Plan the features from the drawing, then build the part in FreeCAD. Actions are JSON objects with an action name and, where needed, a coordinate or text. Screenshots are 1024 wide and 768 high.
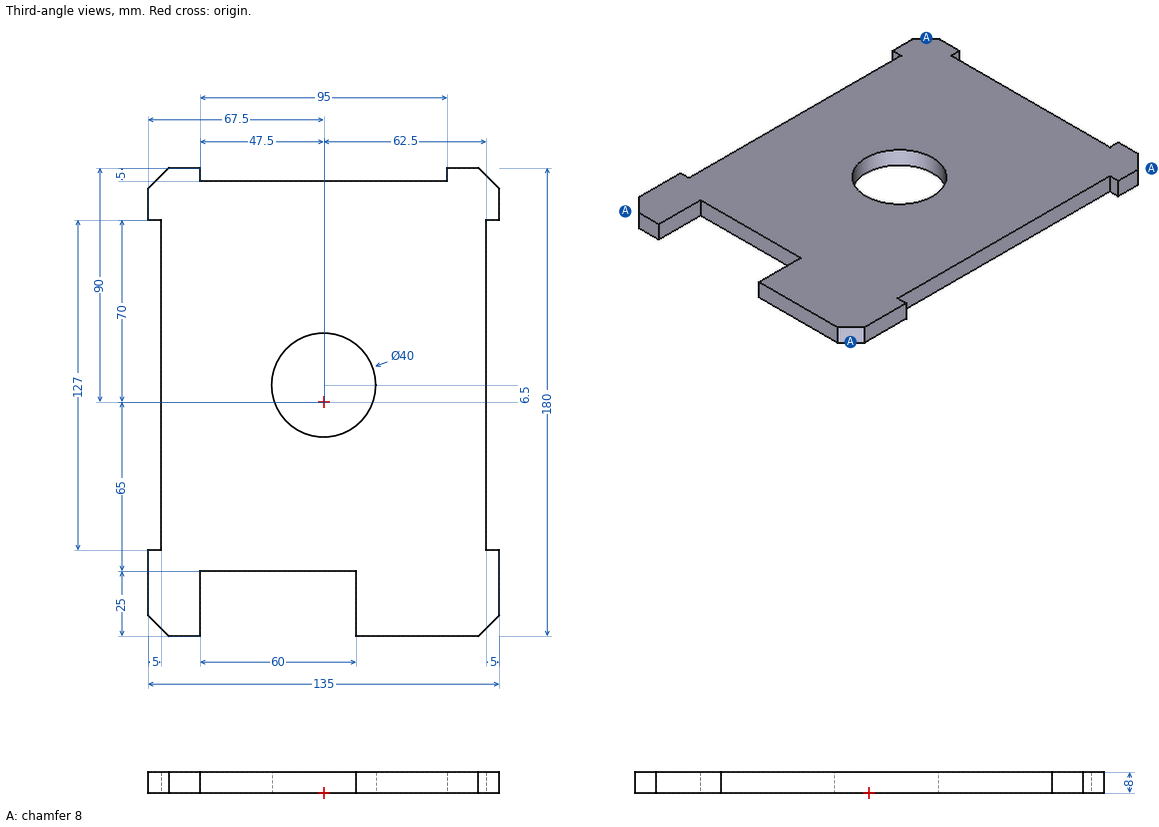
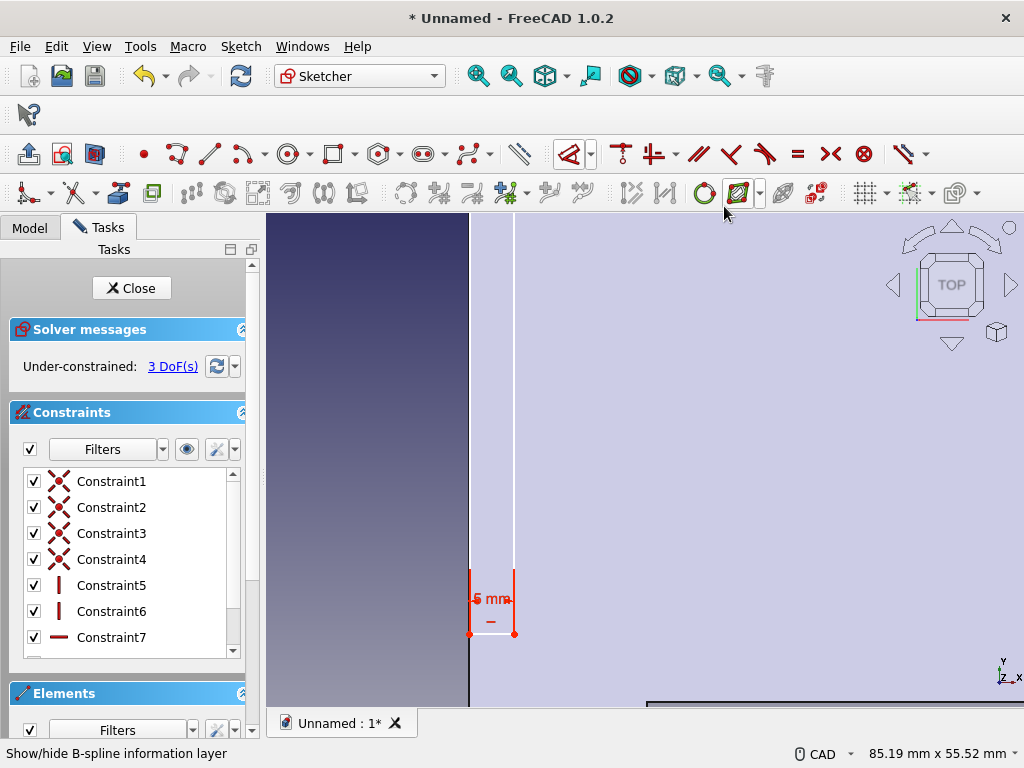
{"action": "scroll", "coordinate": [493, 630], "scroll_direction": "down", "scroll_amount": 6}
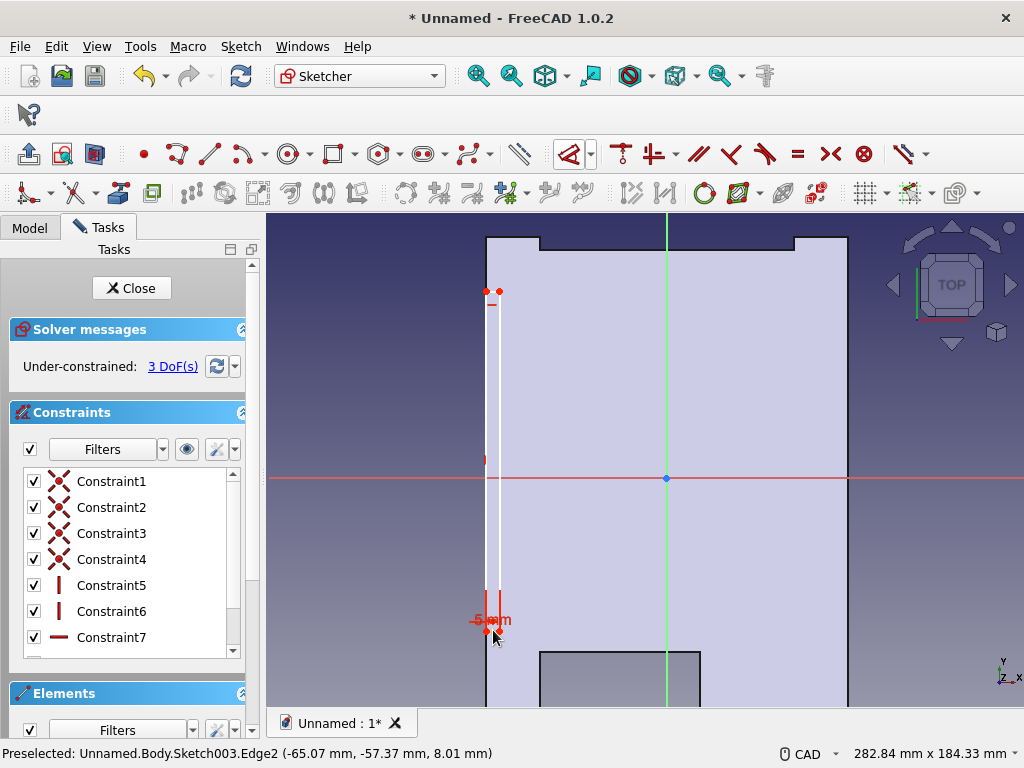
{"action": "left_click", "coordinate": [486, 530]}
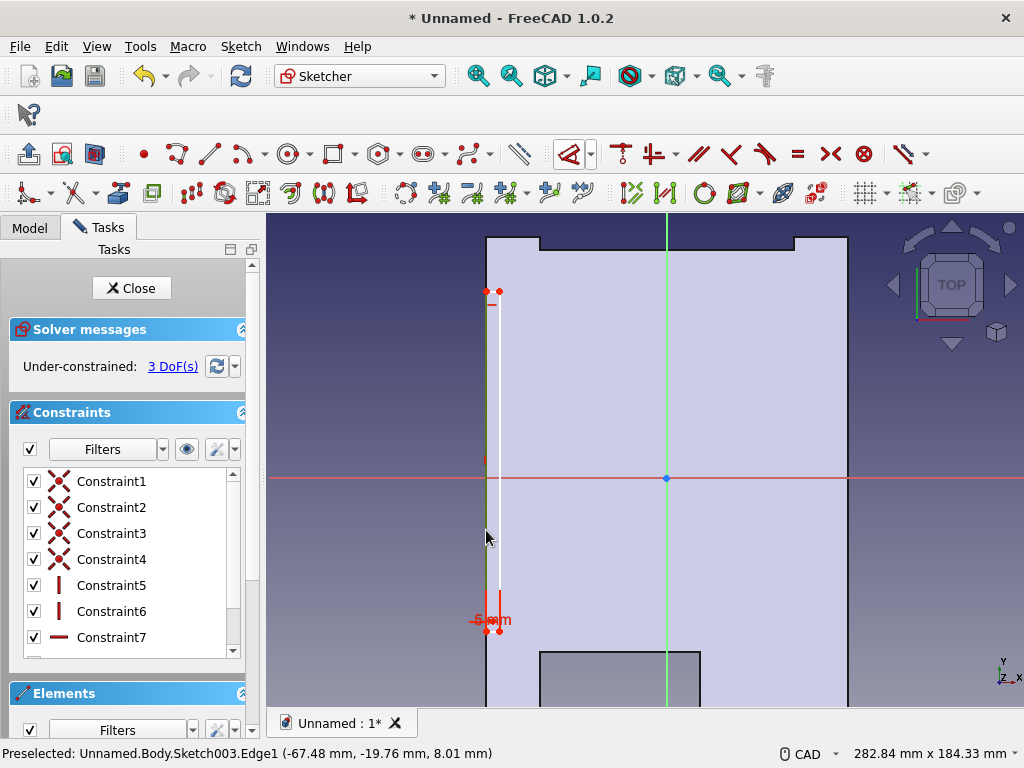
{"action": "key", "text": "i"}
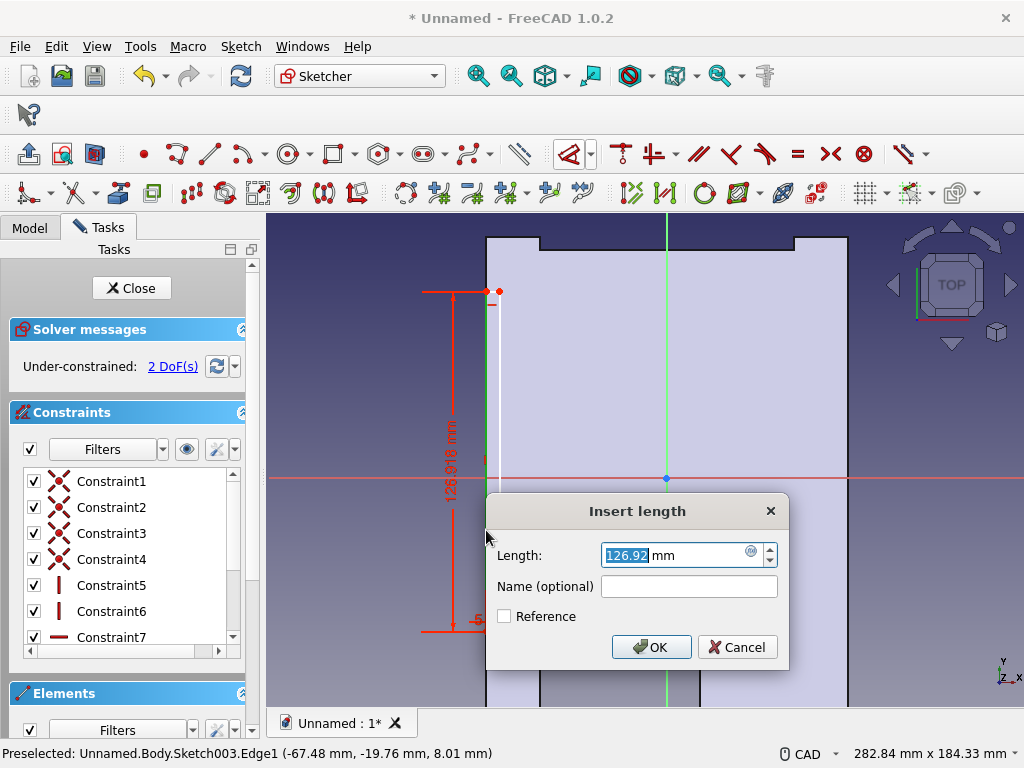
{"action": "type", "text": "127"}
{"action": "key", "text": "Return"}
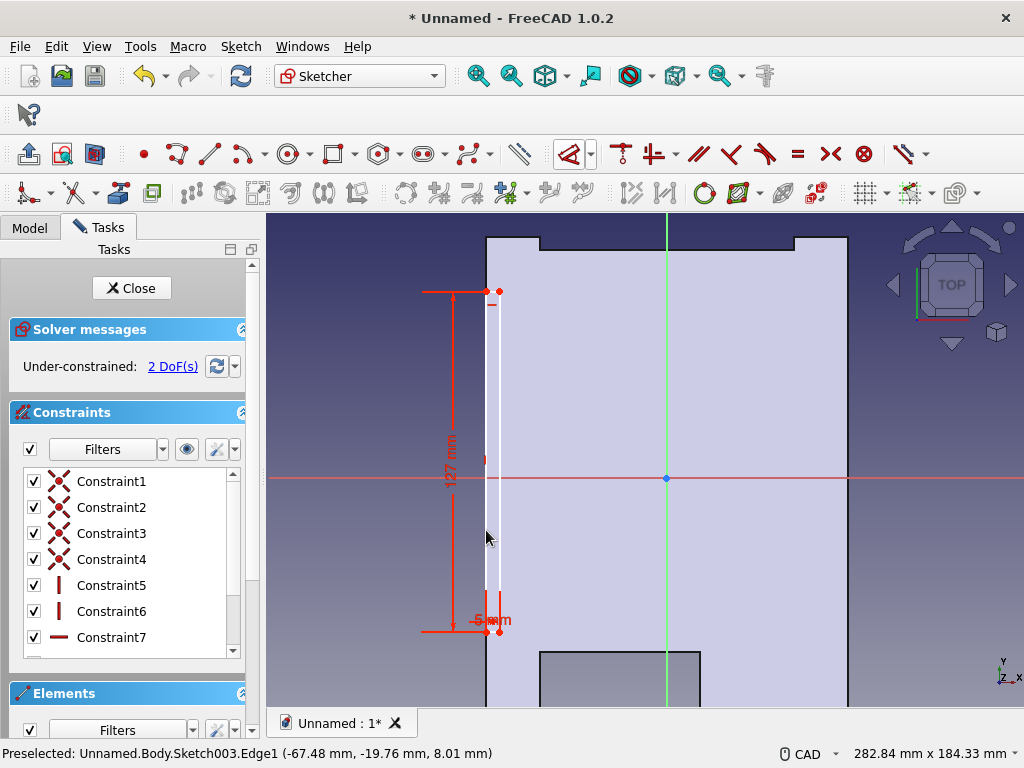
{"action": "left_click", "coordinate": [486, 292]}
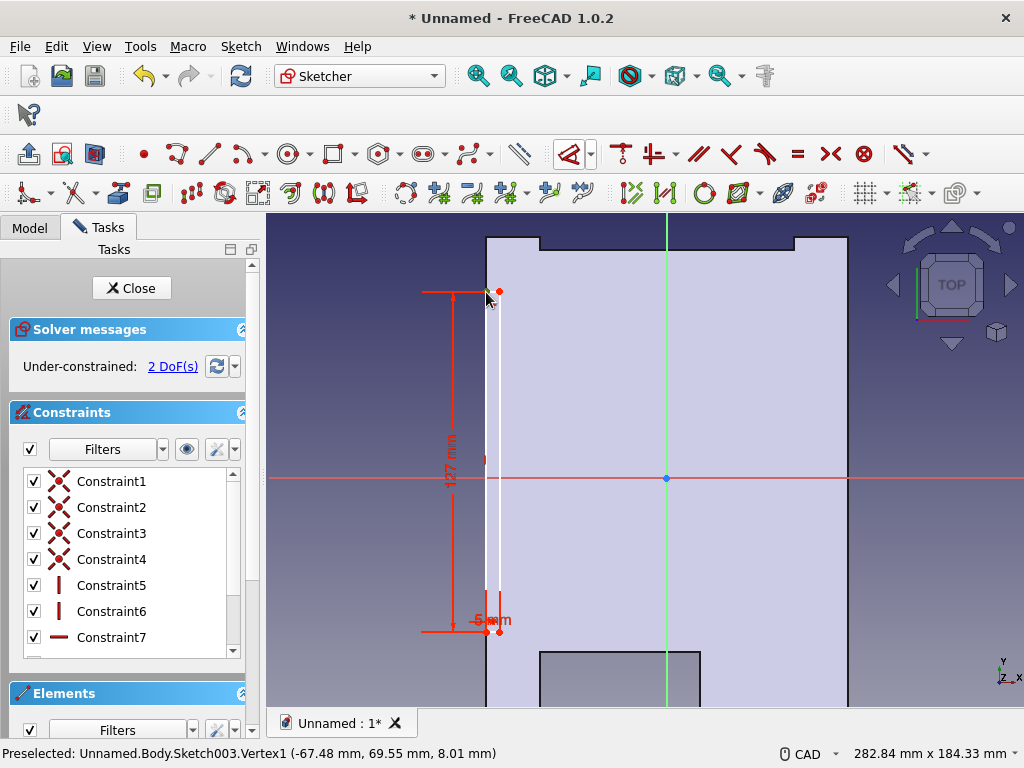
{"action": "left_click", "coordinate": [590, 154]}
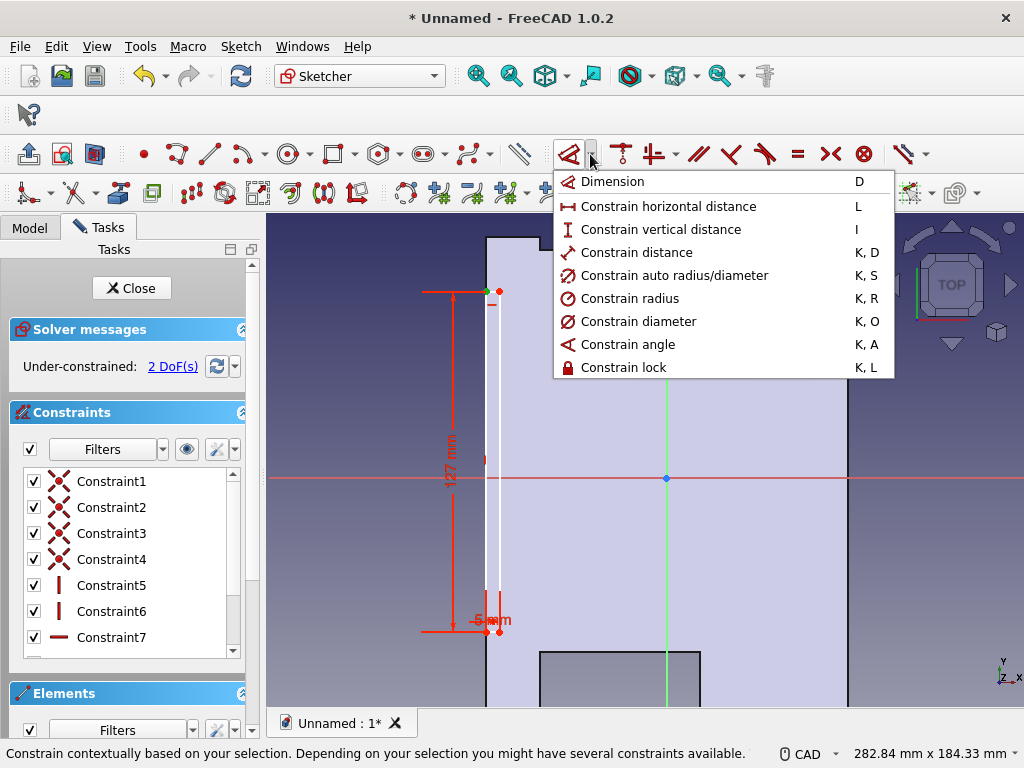
{"action": "left_click", "coordinate": [724, 230]}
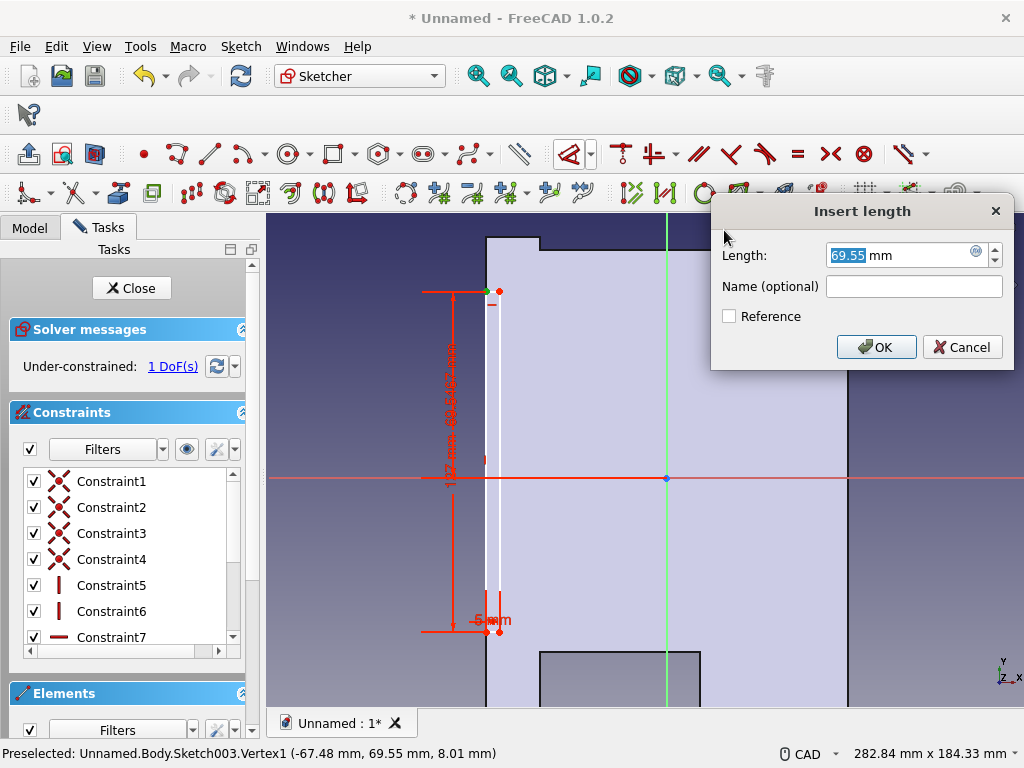
{"action": "type", "text": "70"}
{"action": "key", "text": "Return"}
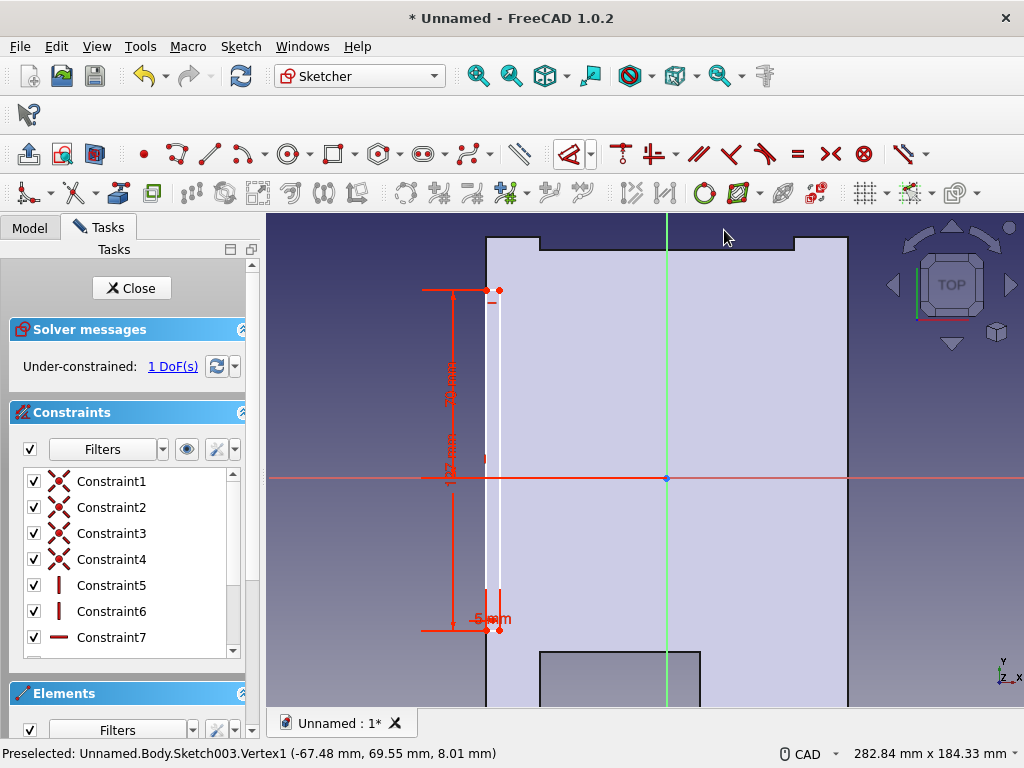
{"action": "left_click", "coordinate": [486, 290]}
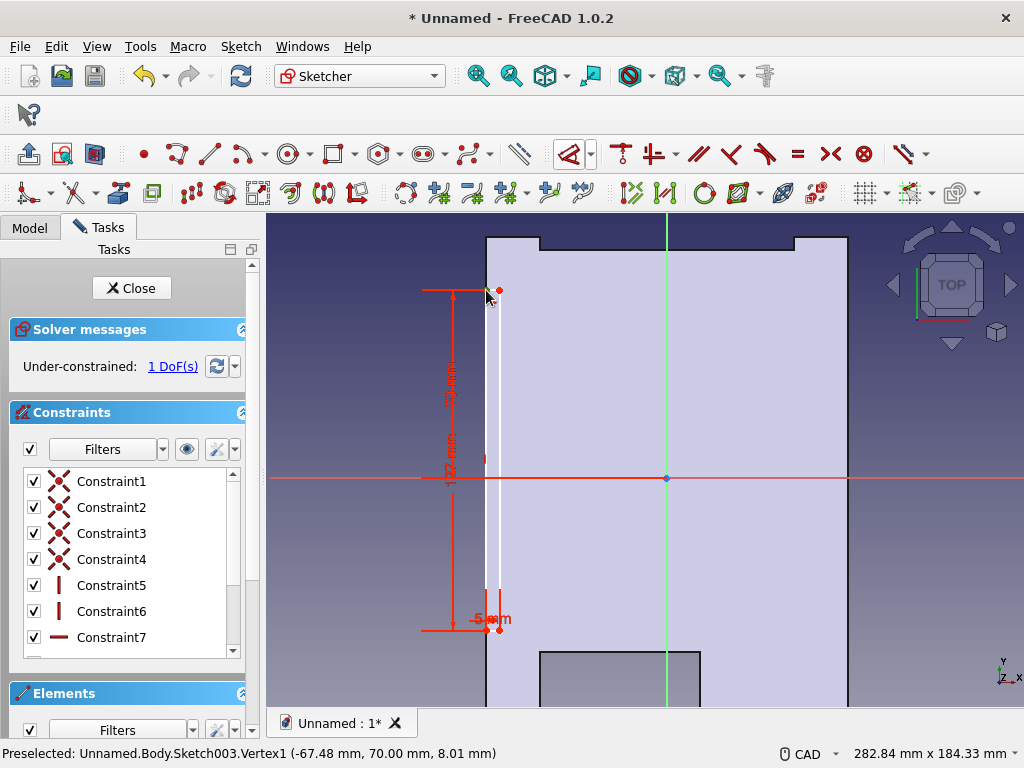
{"action": "key", "text": "l"}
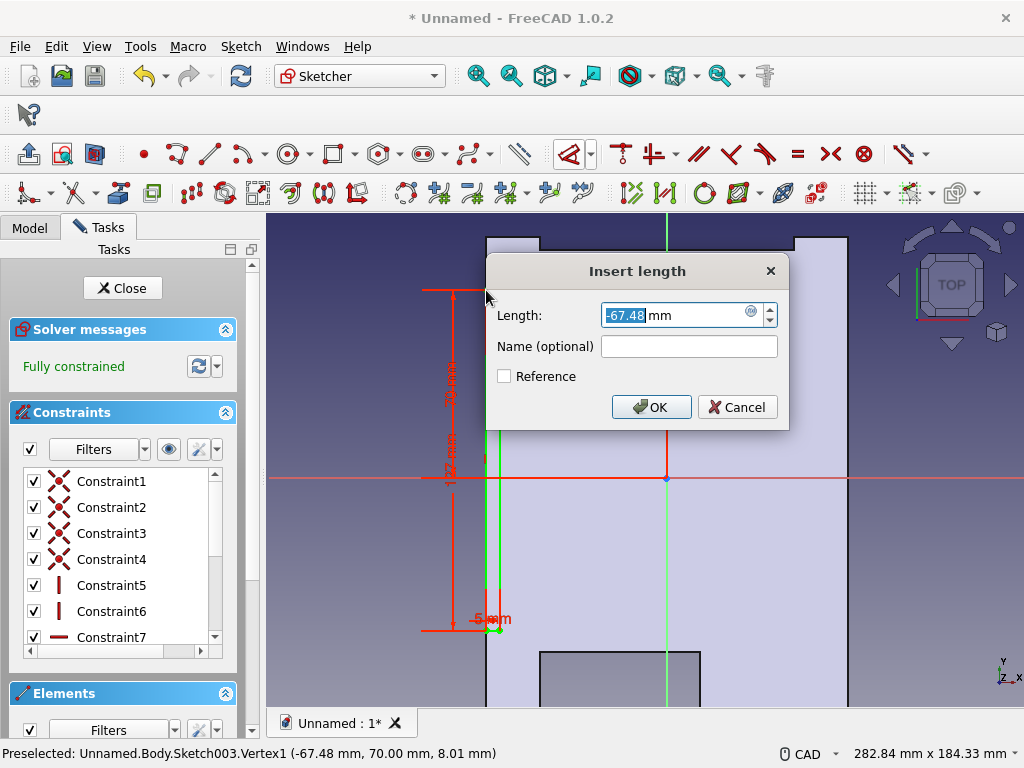
{"action": "type", "text": "-67.5"}
{"action": "key", "text": "Return"}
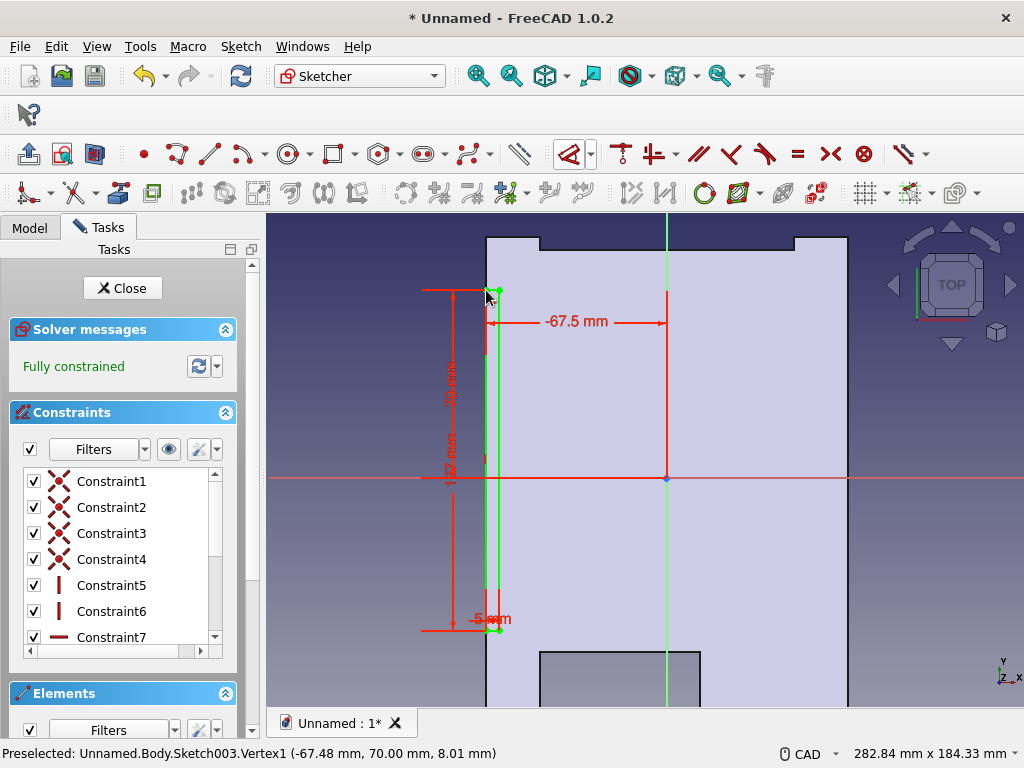
{"action": "left_click", "coordinate": [123, 288]}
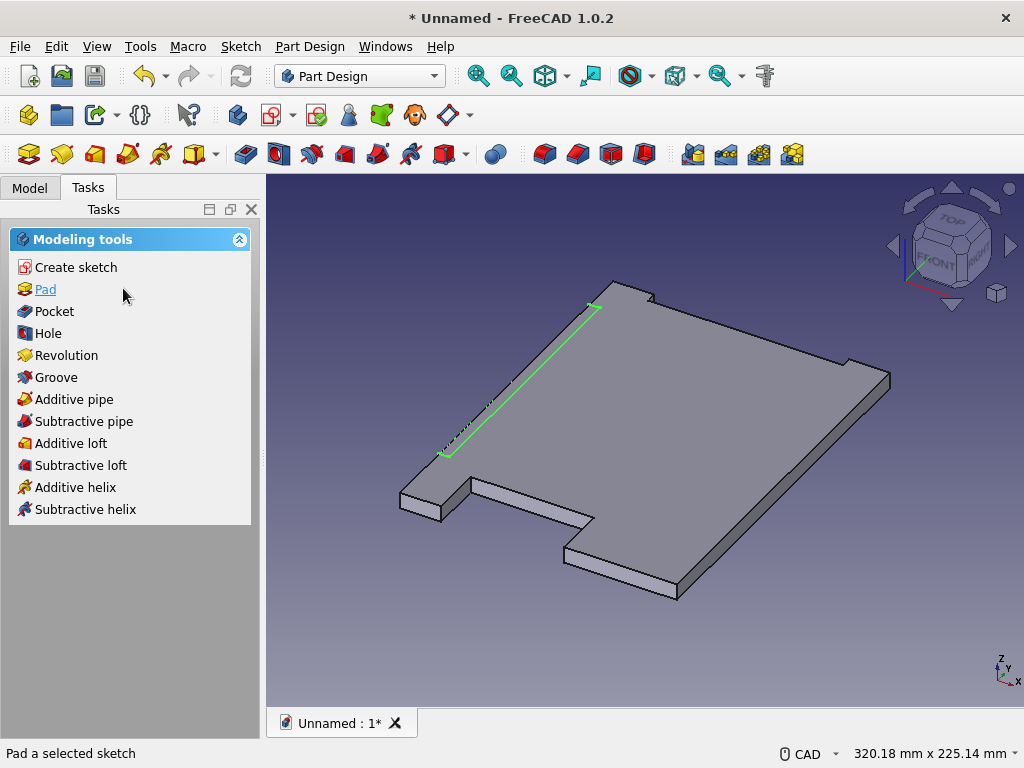
{"action": "left_click", "coordinate": [246, 154]}